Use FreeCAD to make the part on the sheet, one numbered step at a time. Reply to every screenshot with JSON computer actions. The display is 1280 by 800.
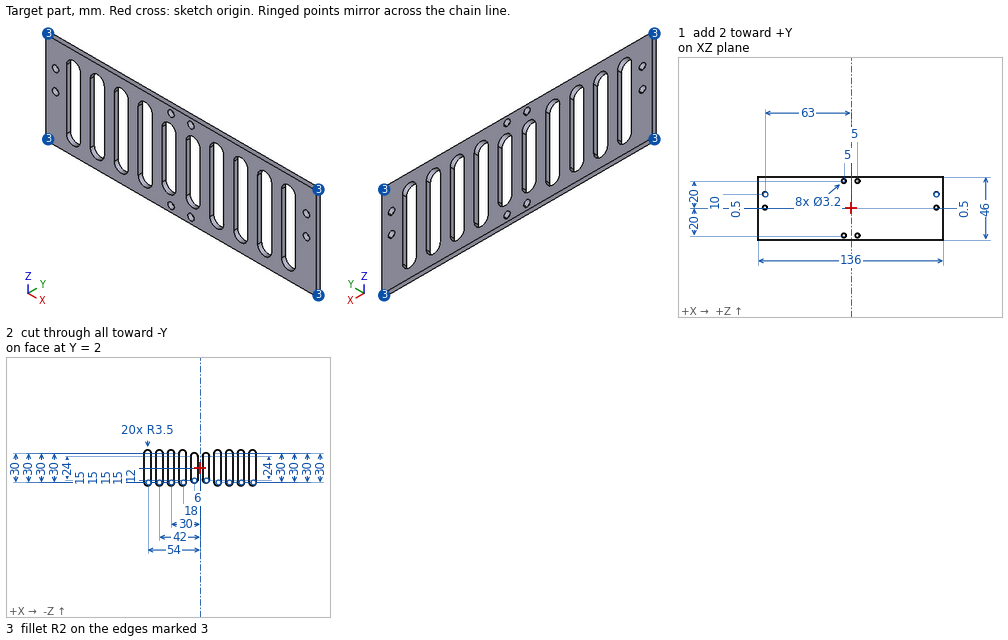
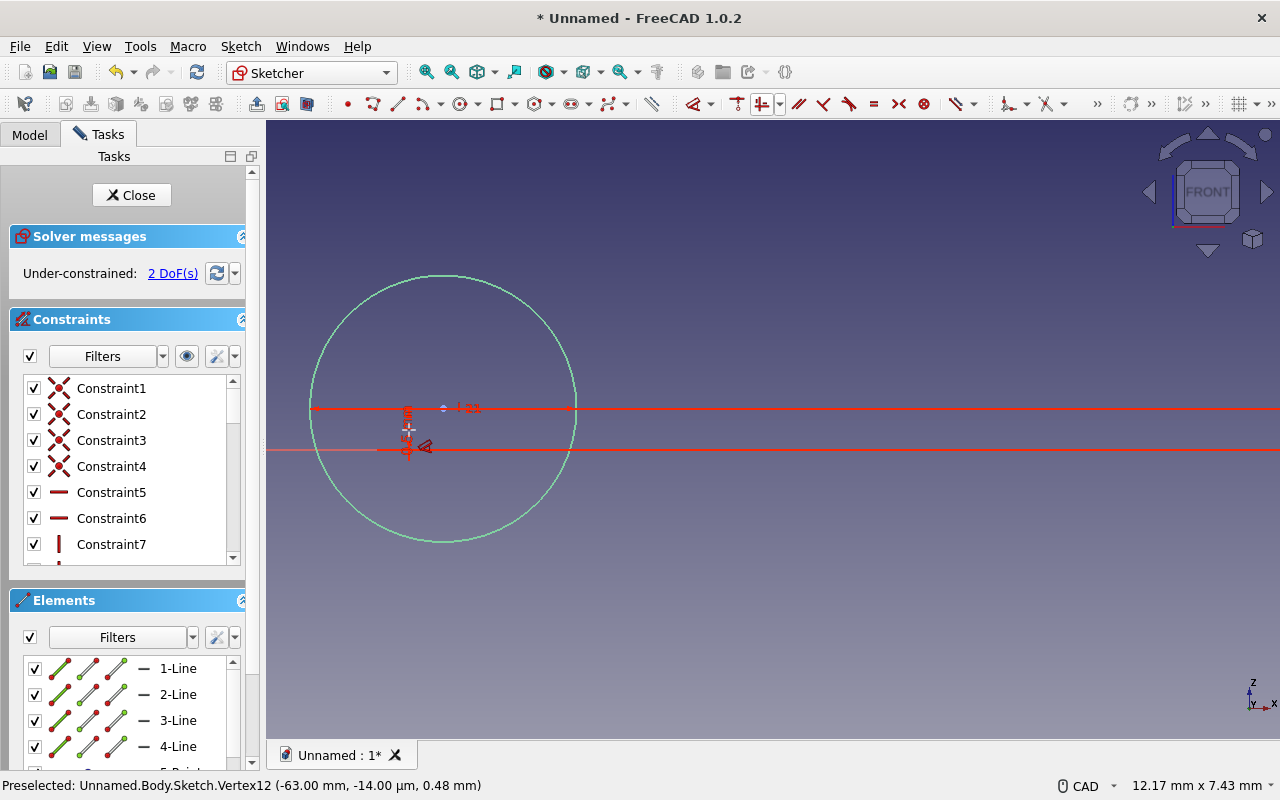
{"action": "scroll", "coordinate": [443, 428], "scroll_direction": "down", "scroll_amount": 15}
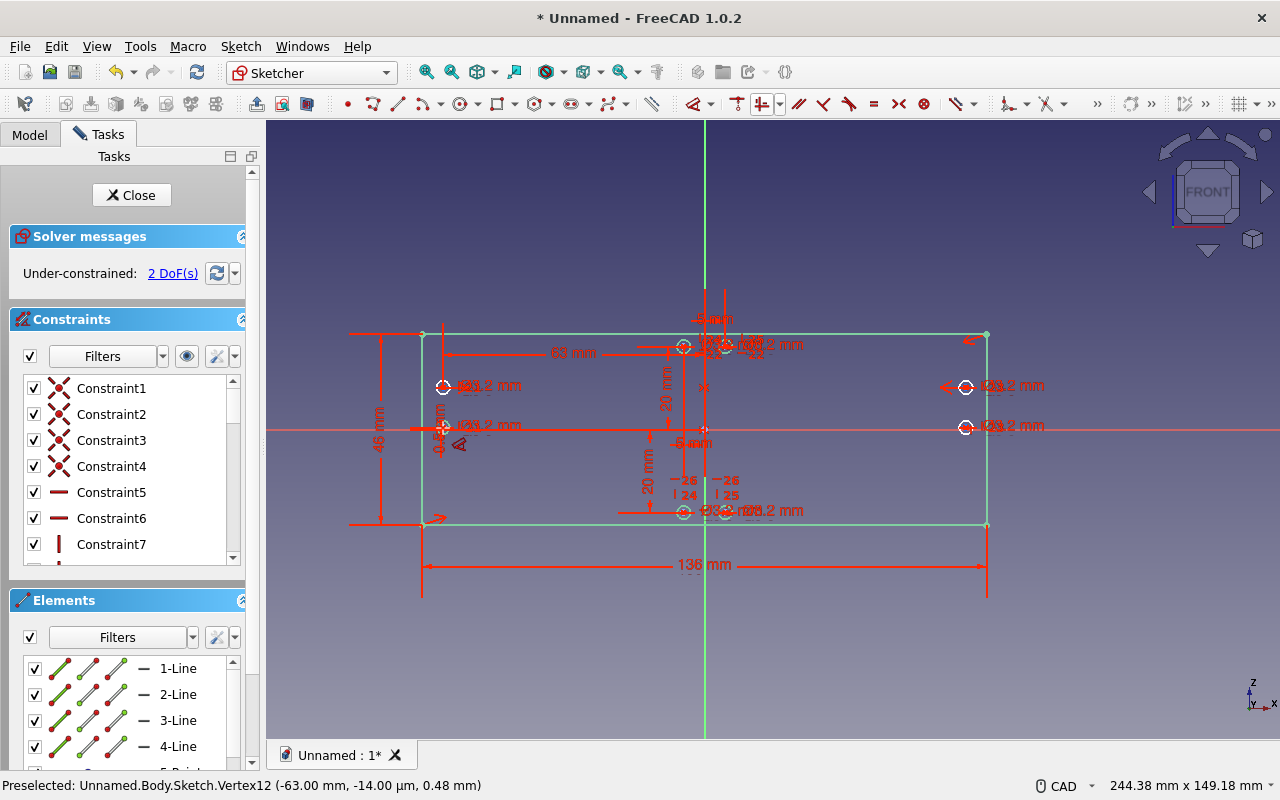
{"action": "scroll", "coordinate": [966, 428], "scroll_direction": "up", "scroll_amount": 15}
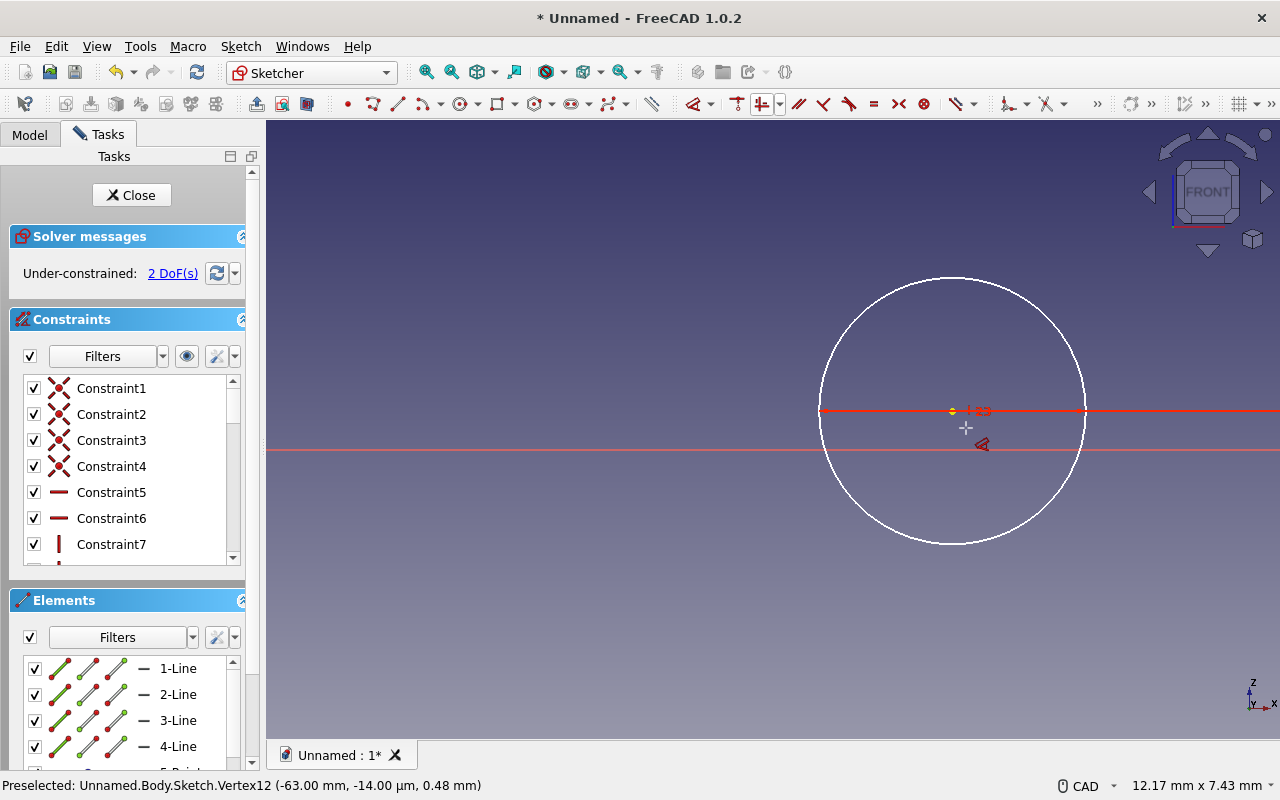
{"action": "left_click", "coordinate": [952, 411]}
{"action": "left_click", "coordinate": [986, 431]}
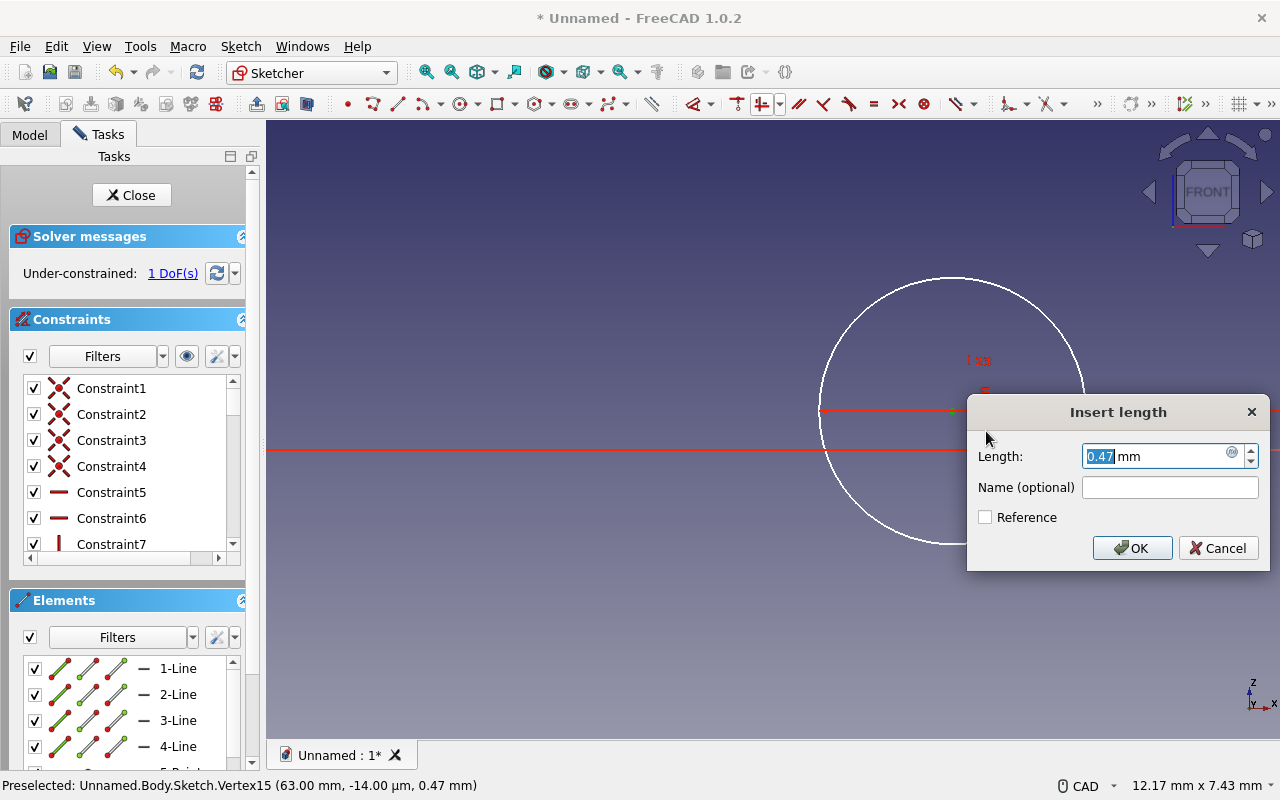
{"action": "type", "text": "0.5"}
{"action": "key", "text": "Return"}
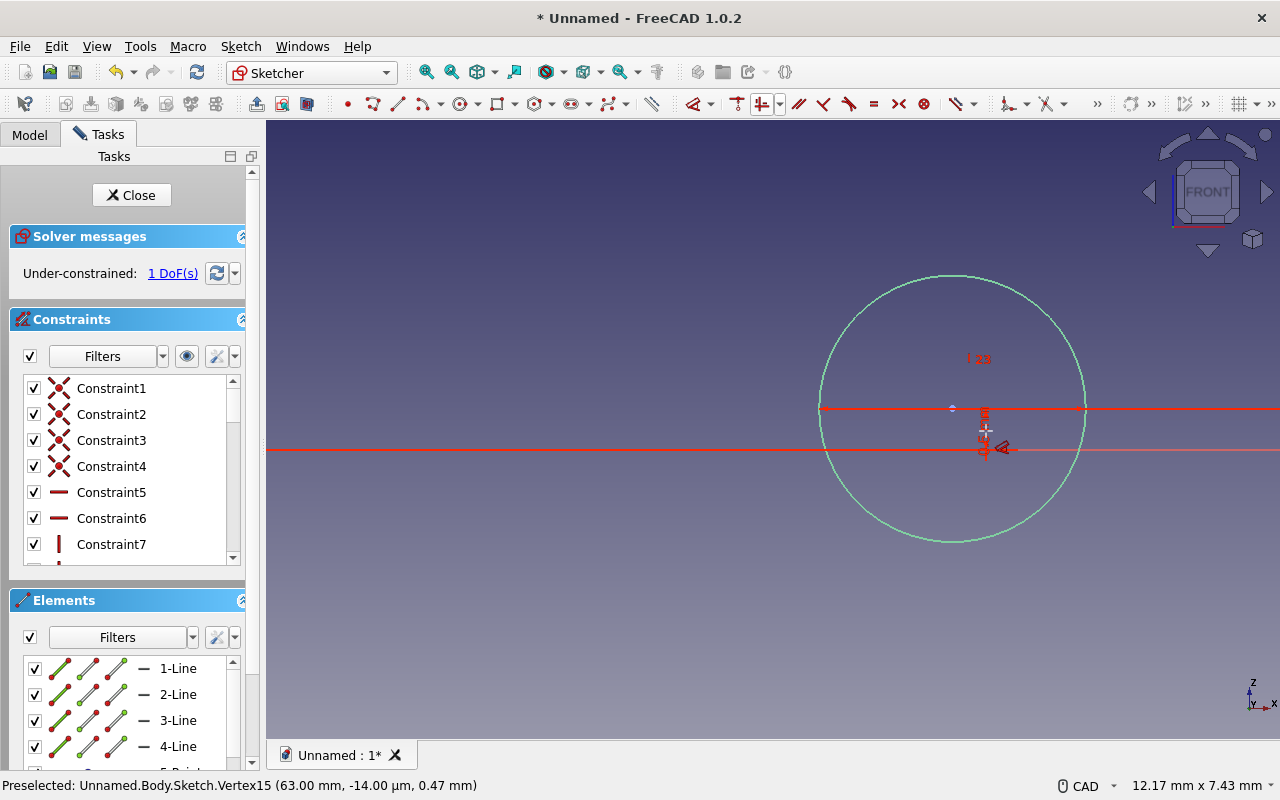
{"action": "scroll", "coordinate": [967, 428], "scroll_direction": "down", "scroll_amount": 15}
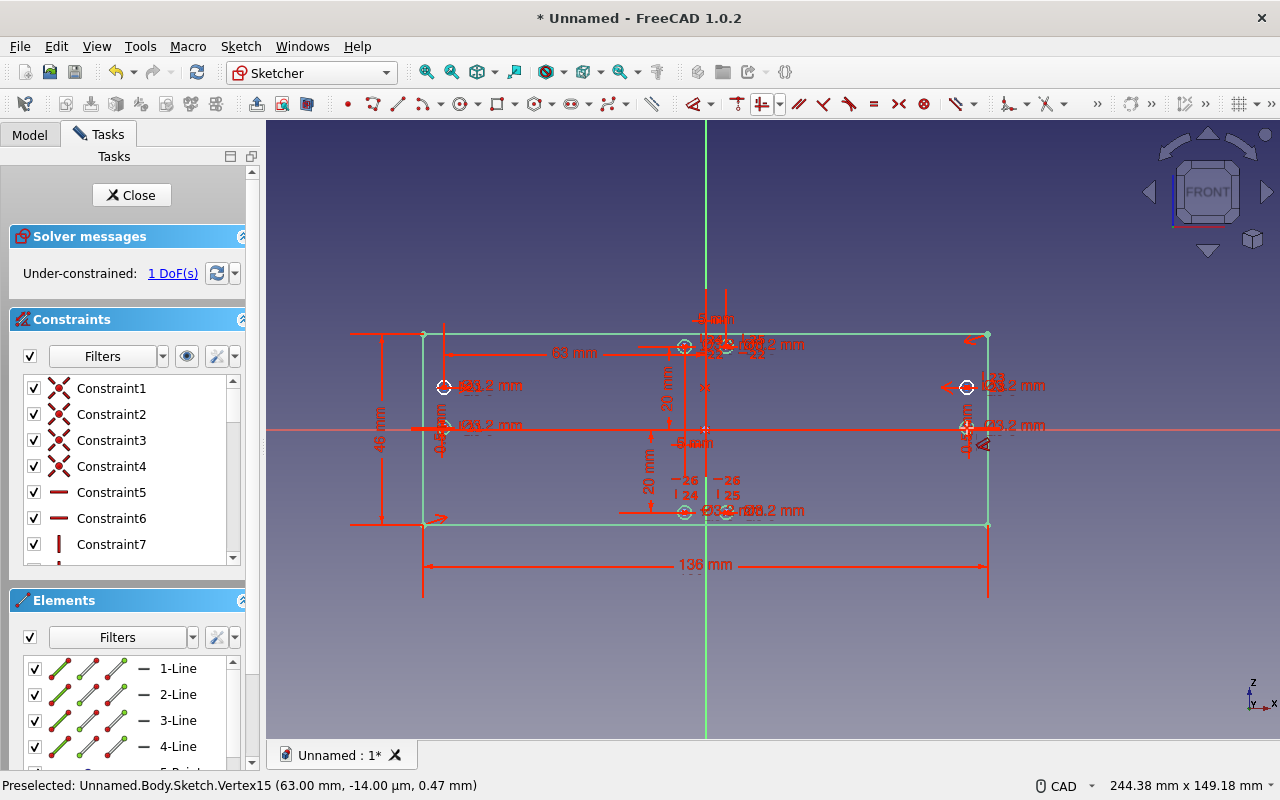
{"action": "left_click", "coordinate": [444, 388]}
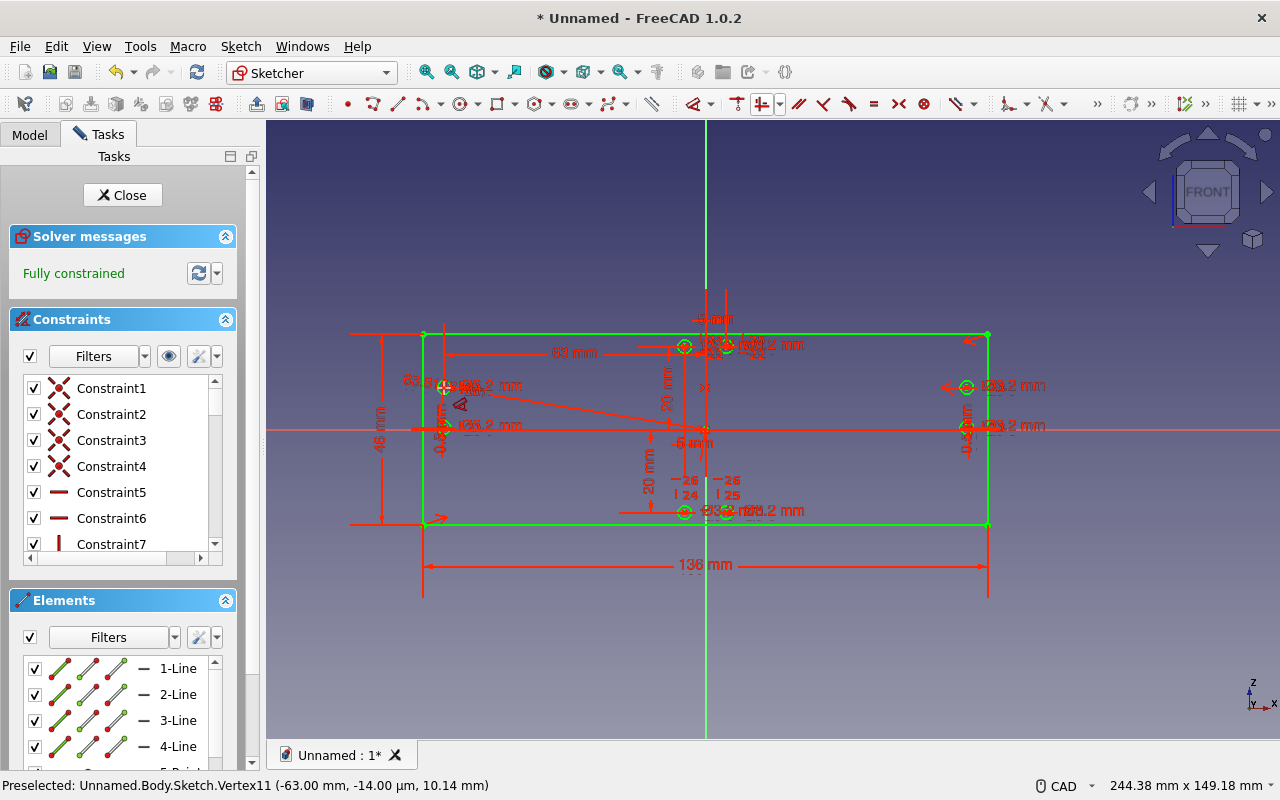
{"action": "left_click", "coordinate": [444, 428]}
{"action": "left_click", "coordinate": [410, 408]}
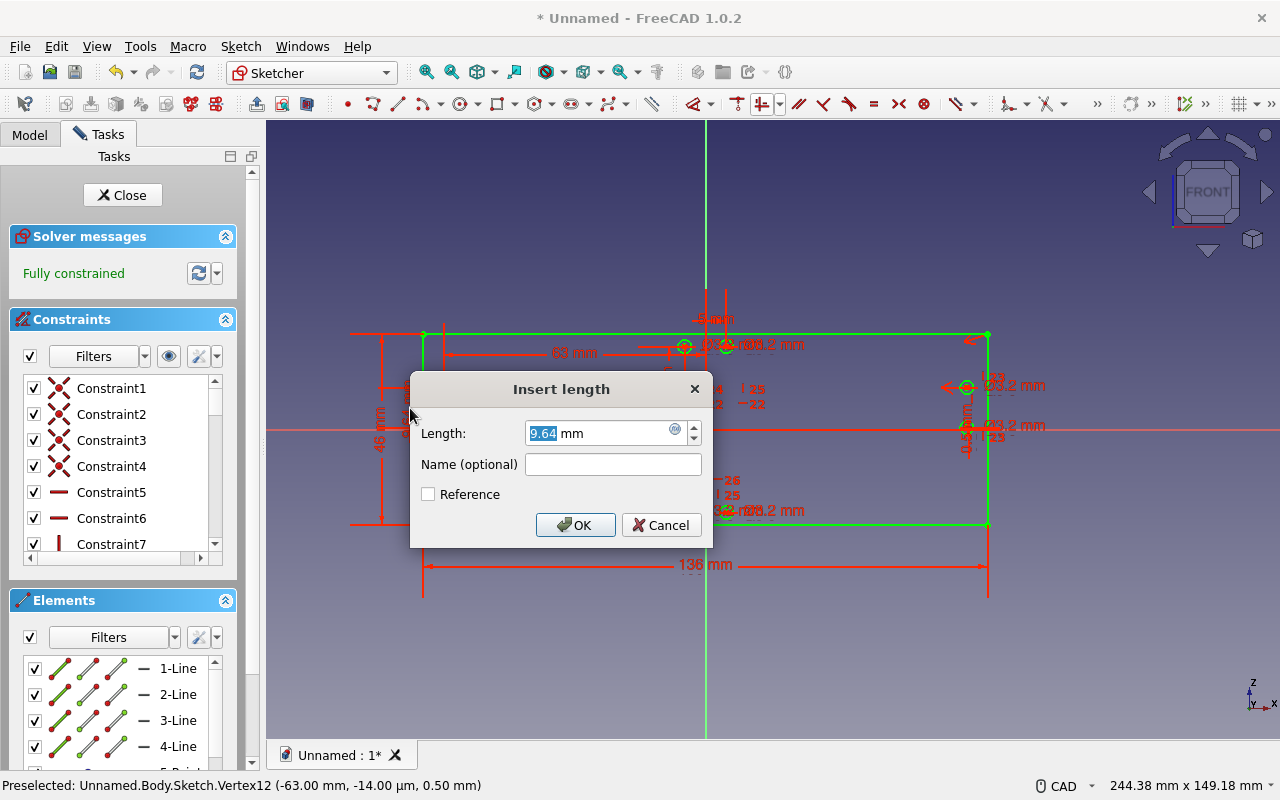
{"action": "type", "text": "10"}
{"action": "key", "text": "Return"}
{"action": "key", "text": "Escape"}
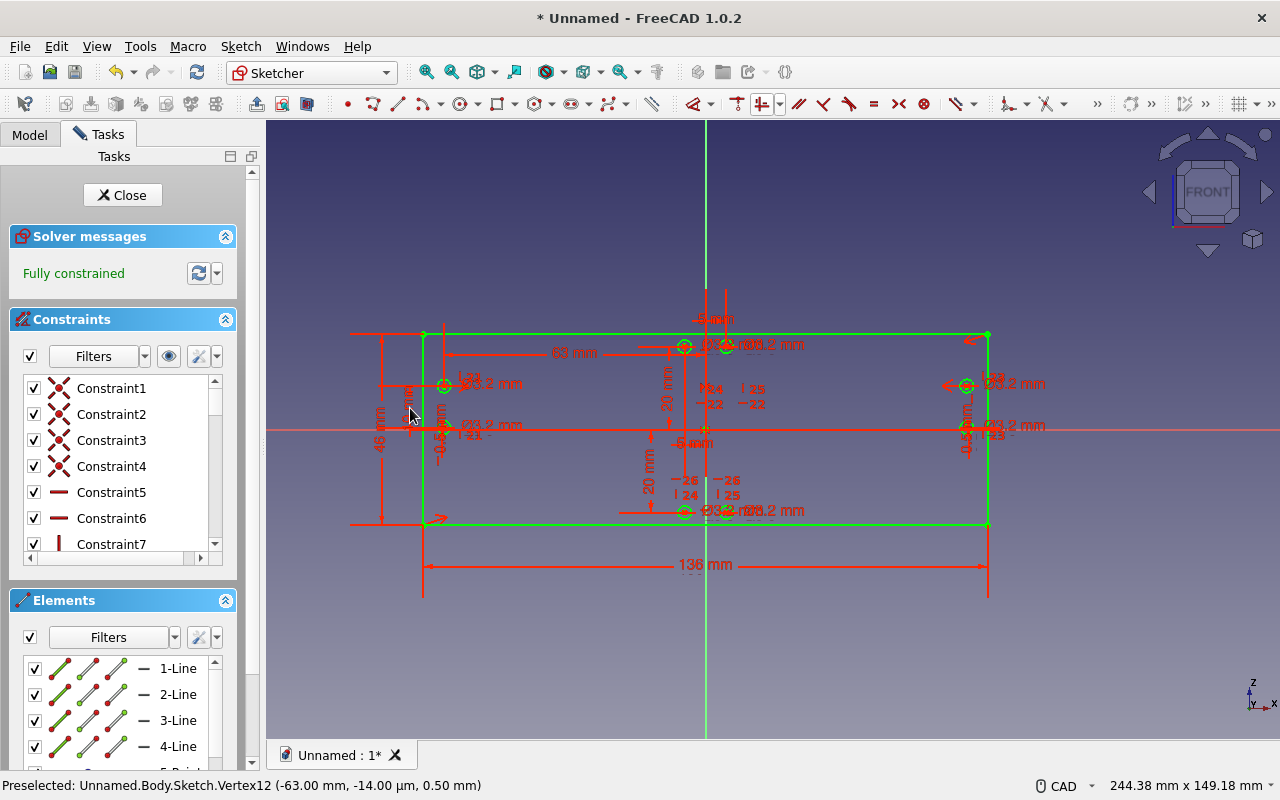
{"action": "left_click", "coordinate": [123, 195]}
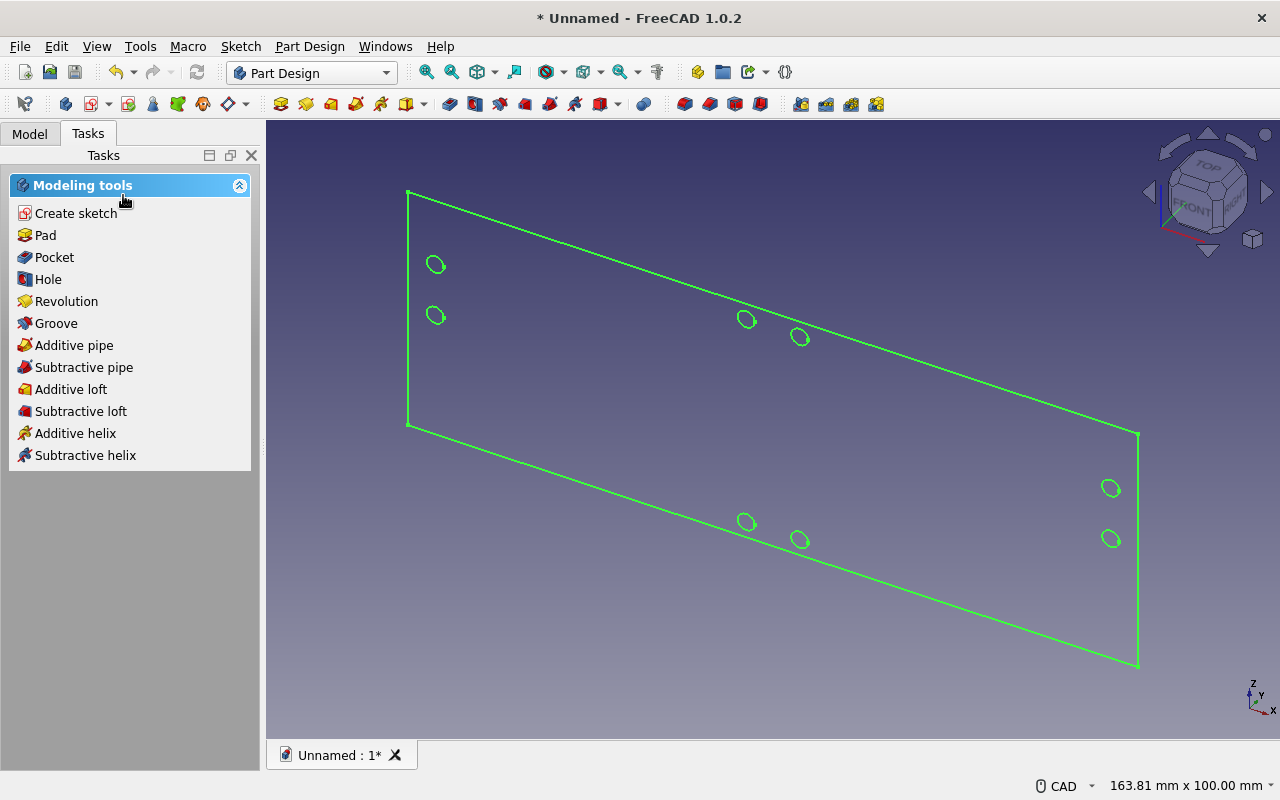
{"action": "left_click", "coordinate": [281, 104]}